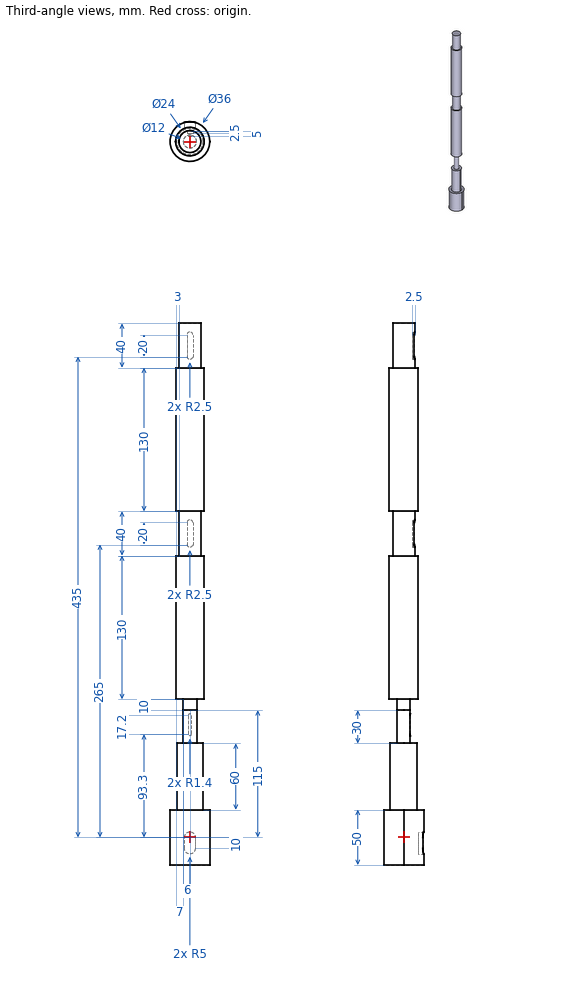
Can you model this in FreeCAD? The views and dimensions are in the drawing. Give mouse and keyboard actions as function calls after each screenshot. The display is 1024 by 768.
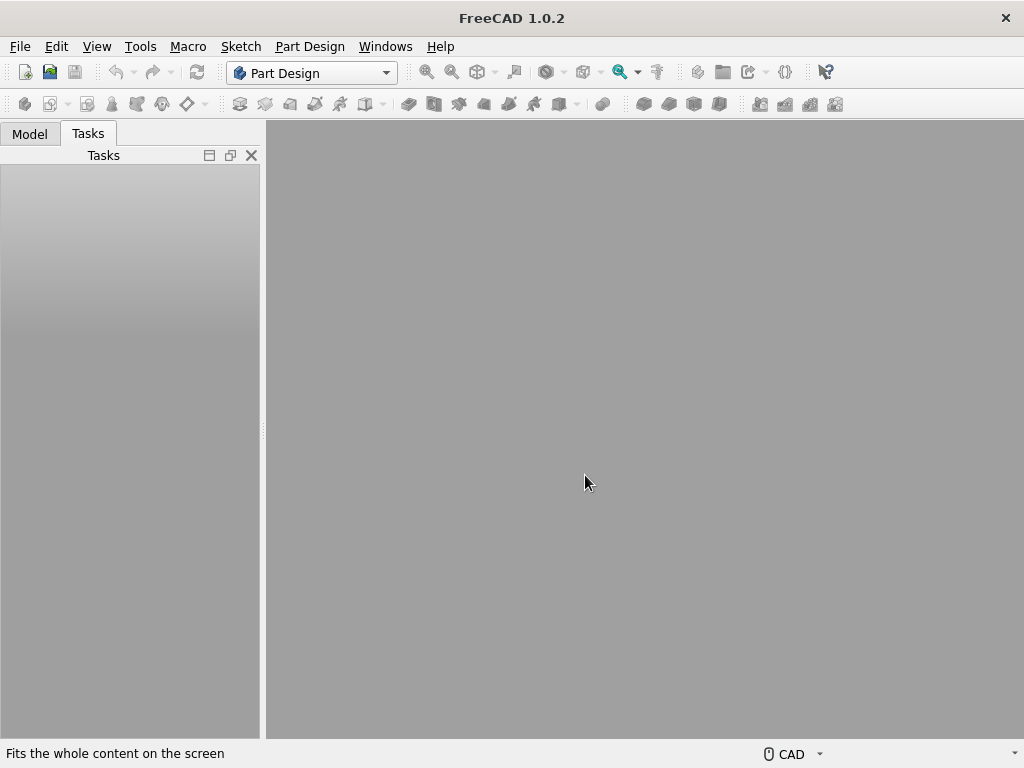
click(25, 72)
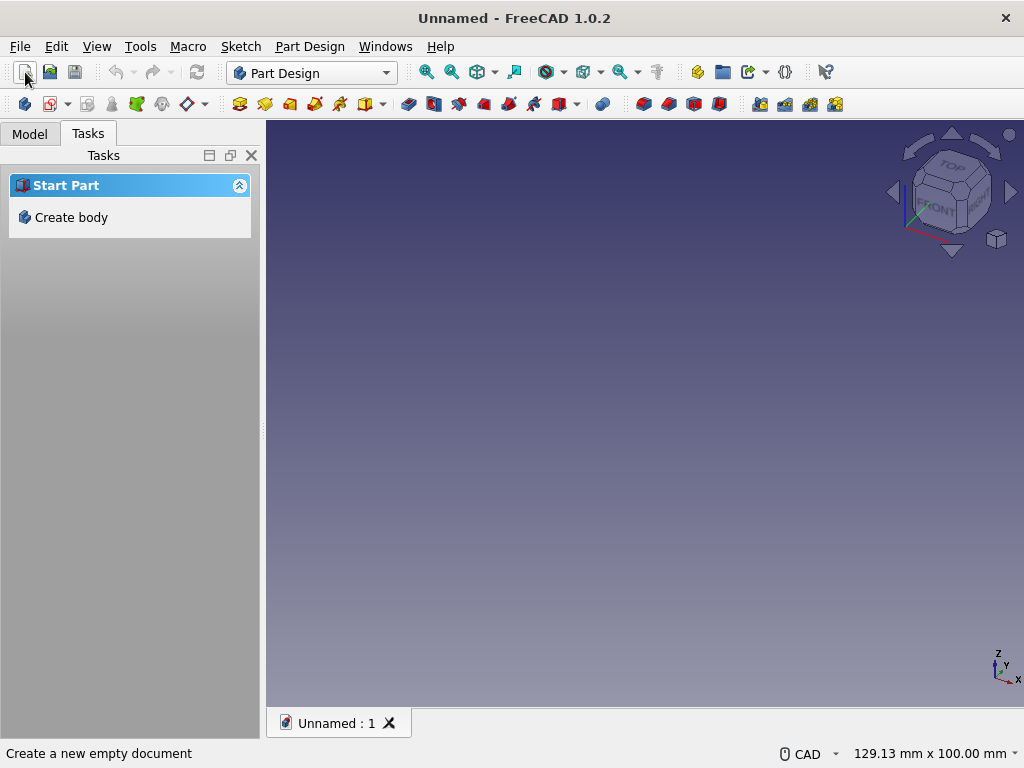
click(50, 104)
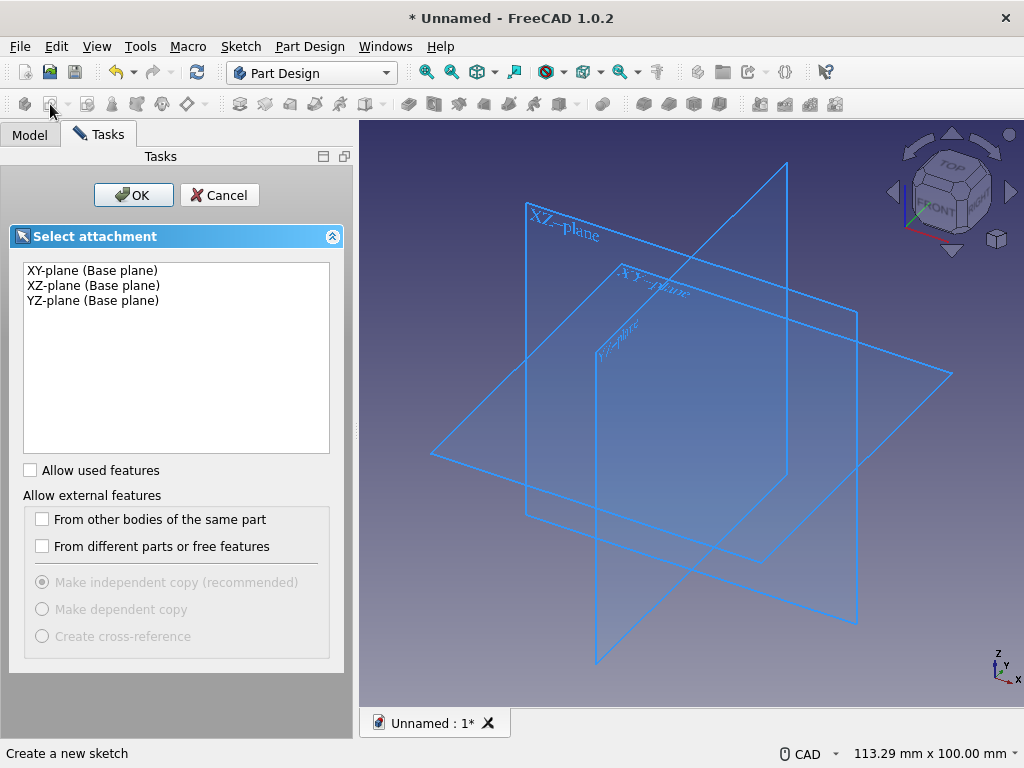
click(84, 270)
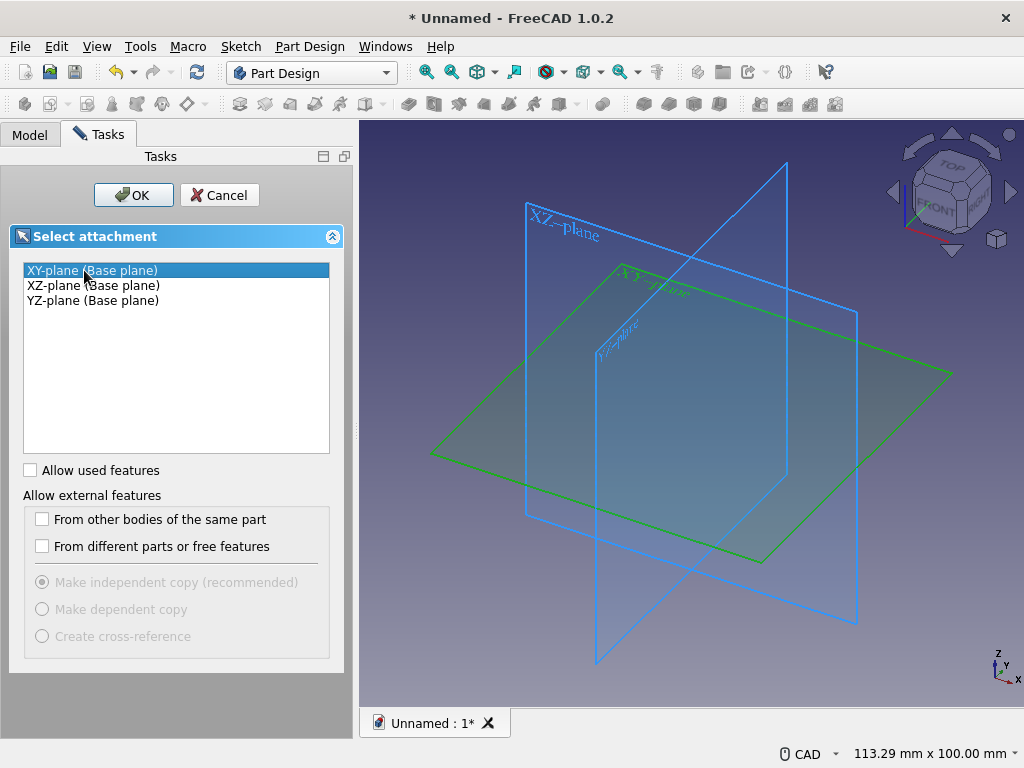
click(134, 195)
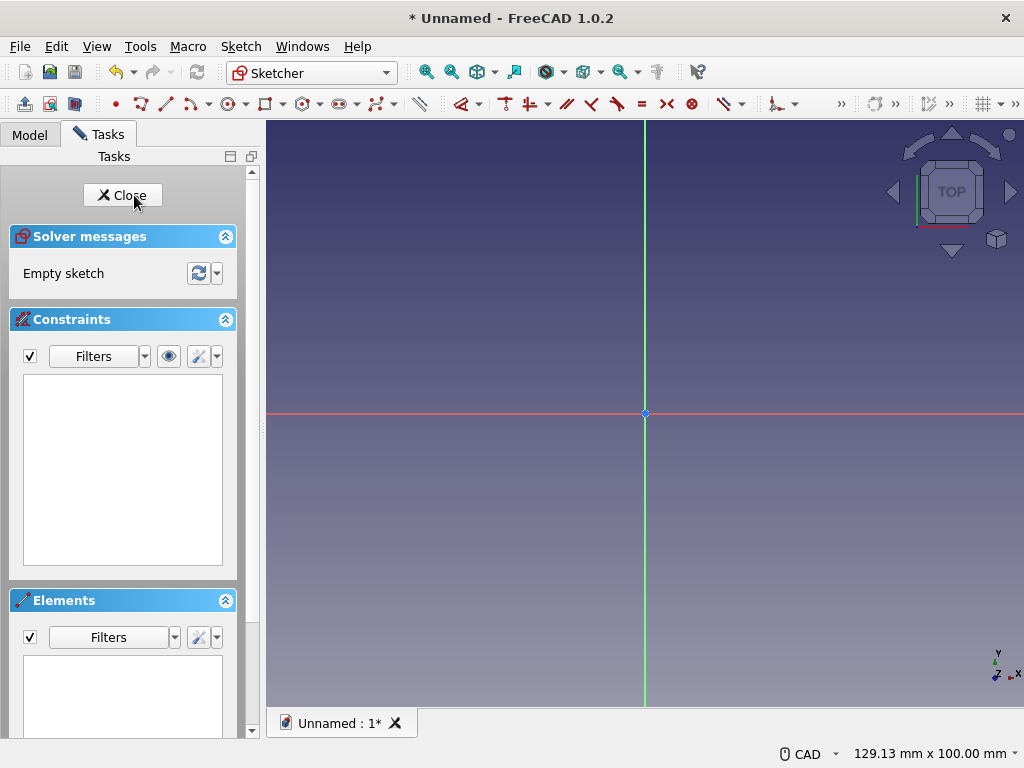
scroll(728, 414, up, 3)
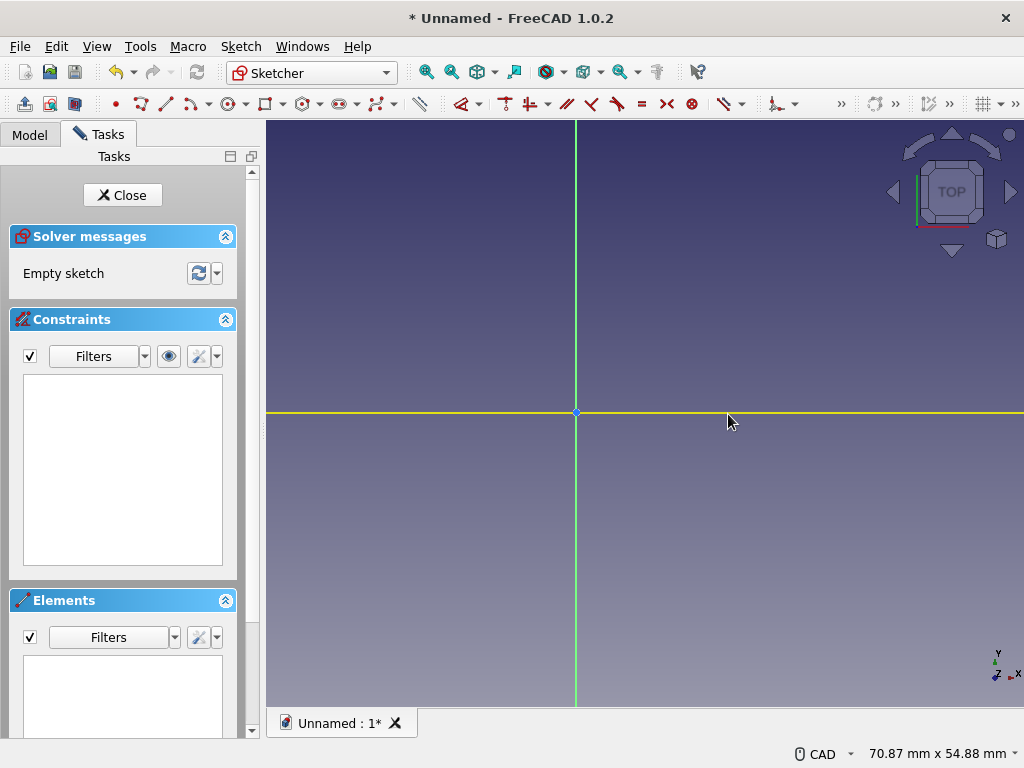
click(228, 104)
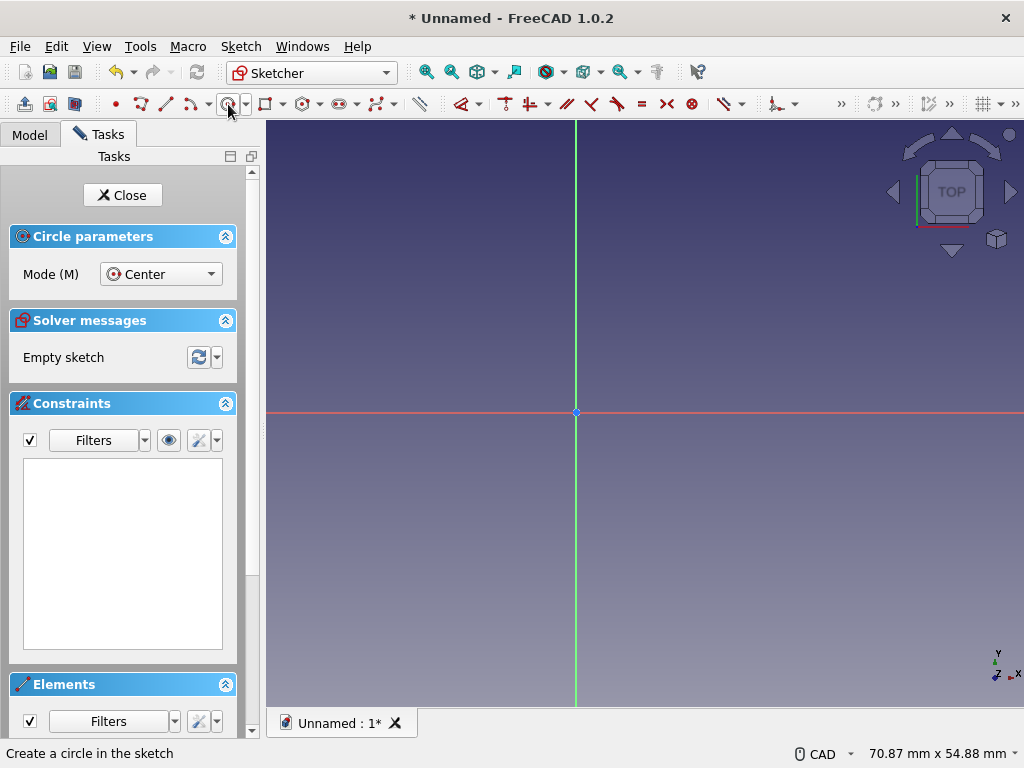
click(576, 413)
click(712, 277)
key(Escape)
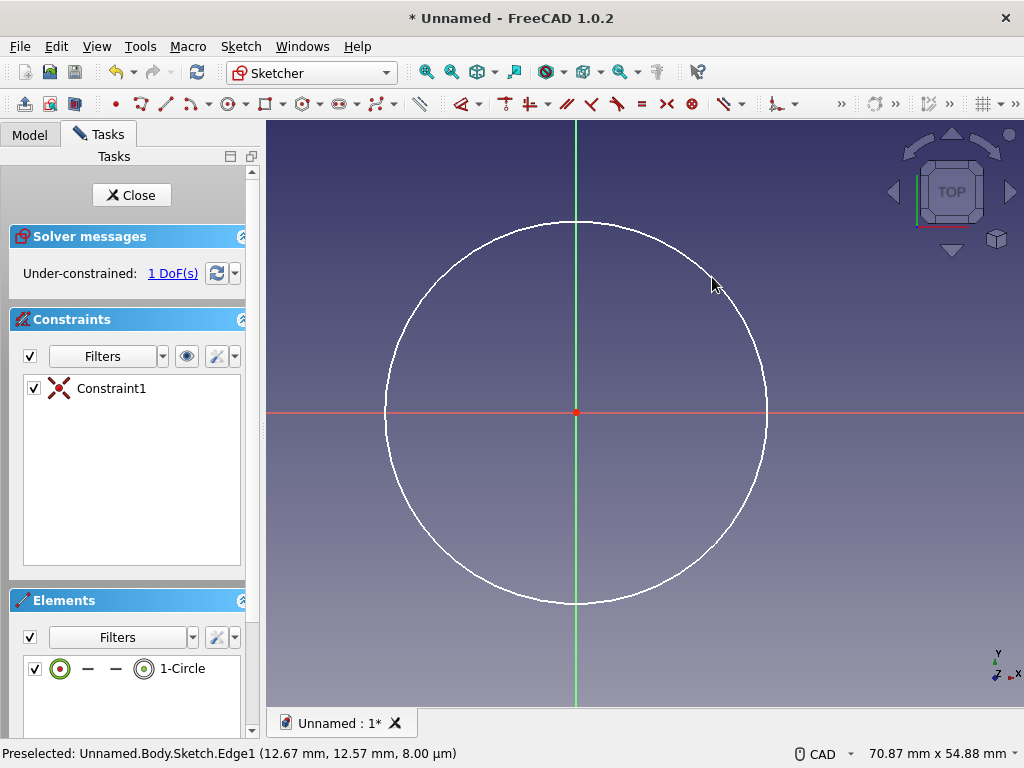
click(460, 104)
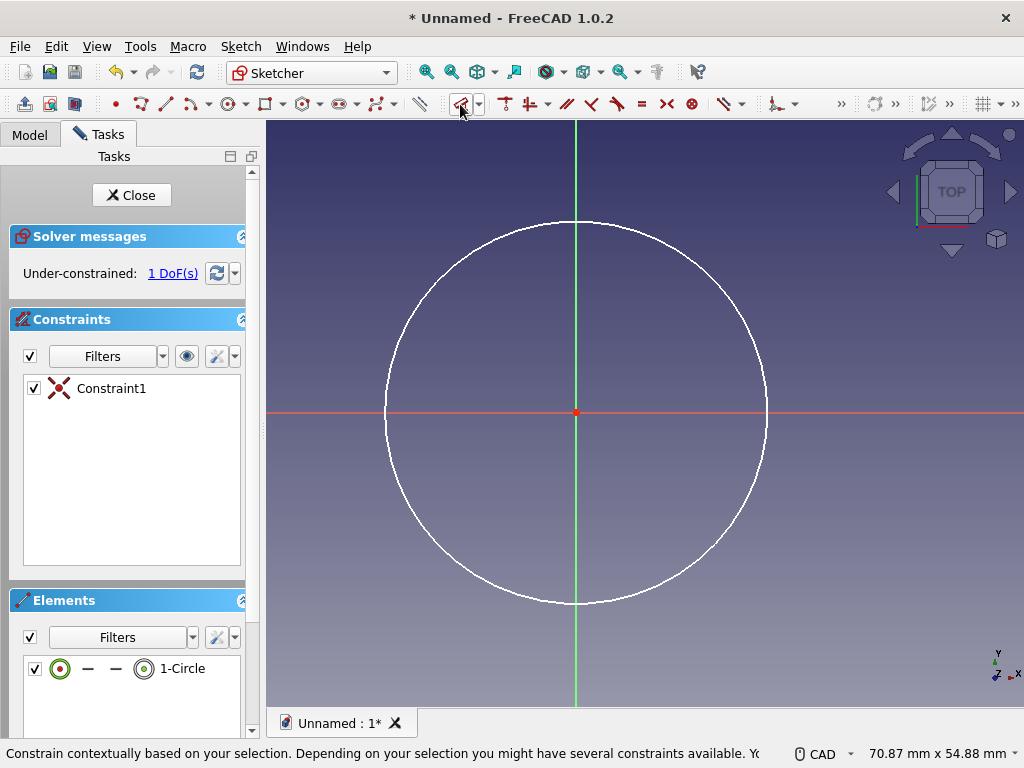
click(711, 277)
click(734, 254)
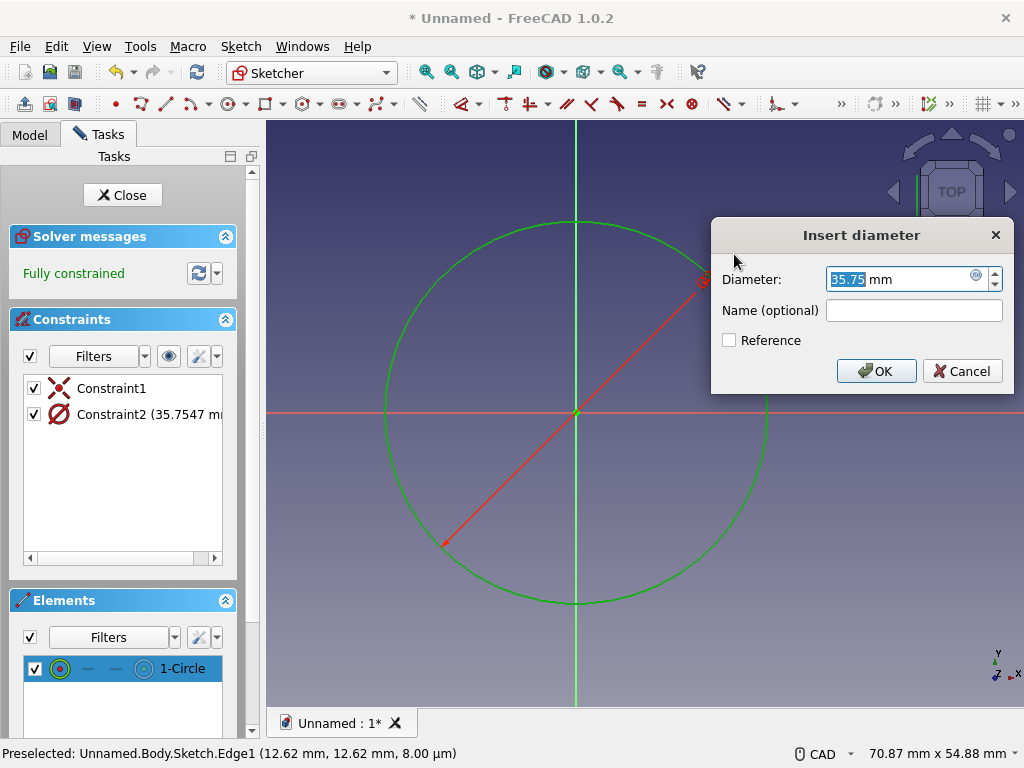
text(36)
key(Return)
key(Escape)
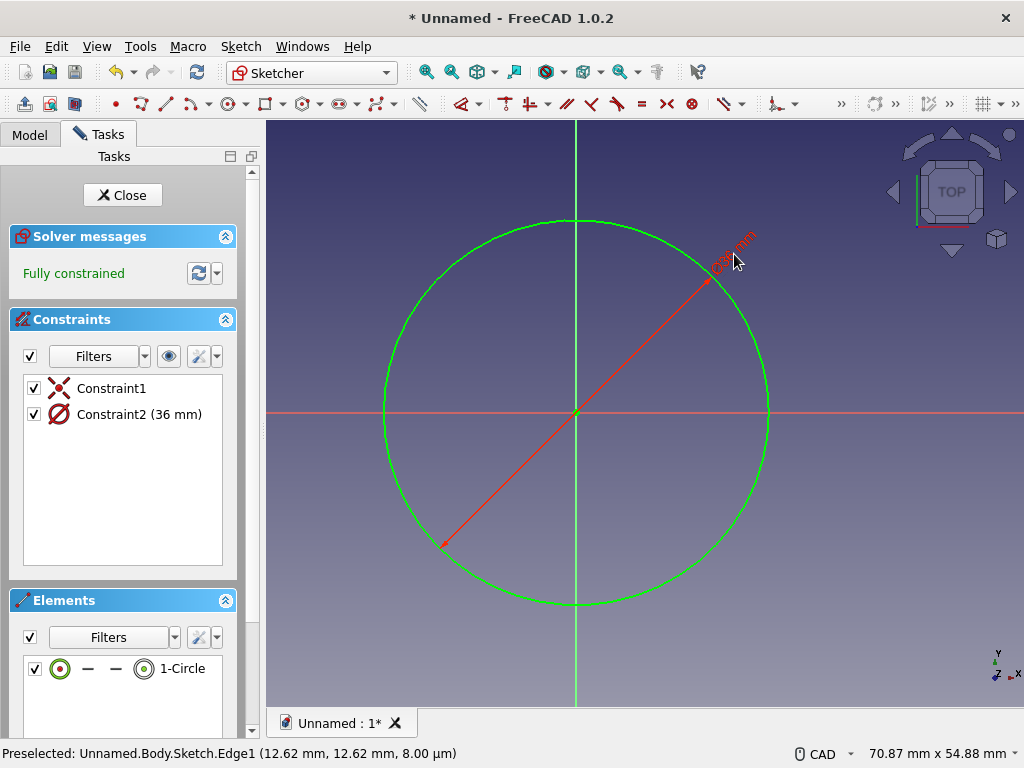
click(123, 195)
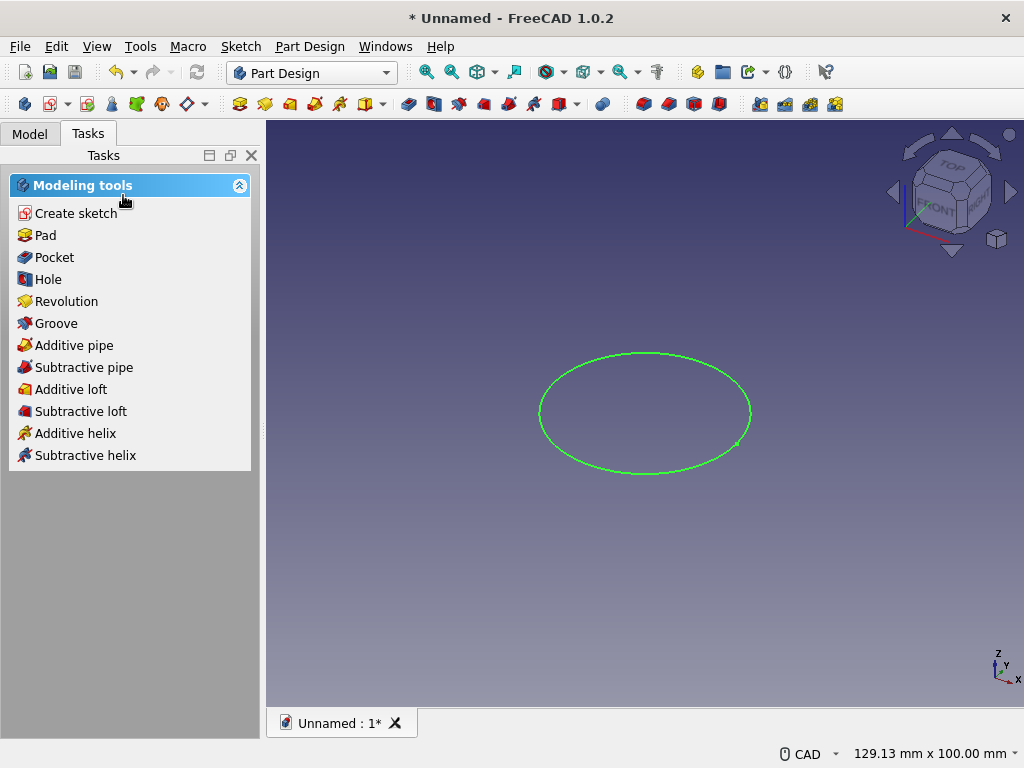
click(240, 104)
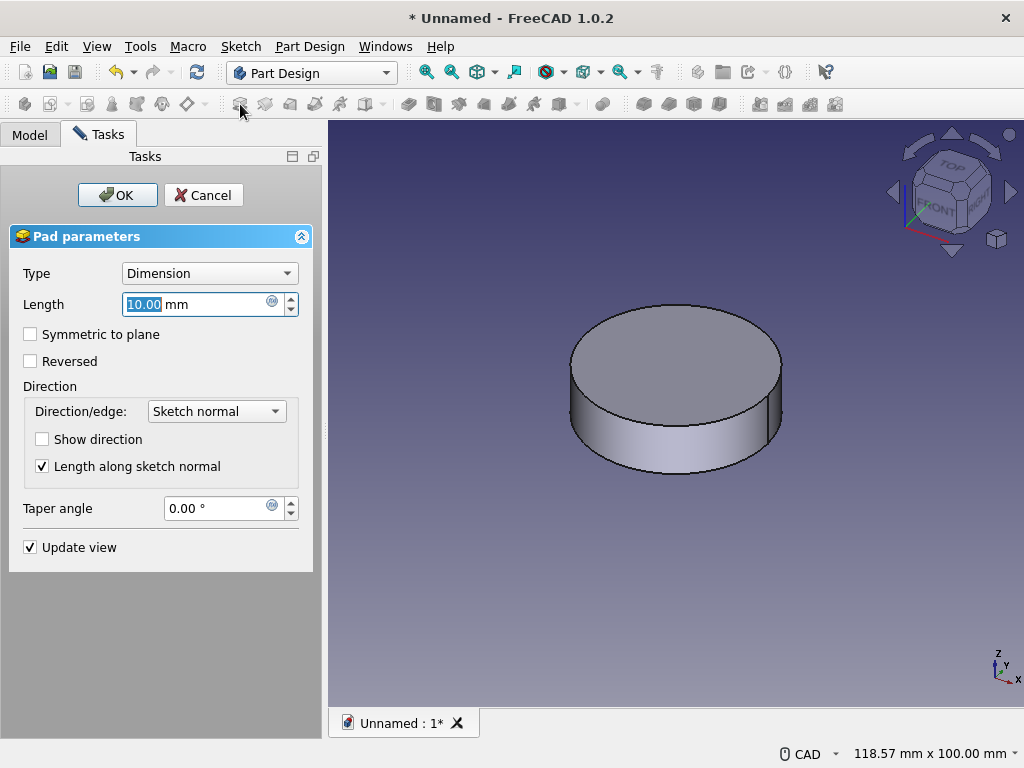
text(50)
key(Tab)